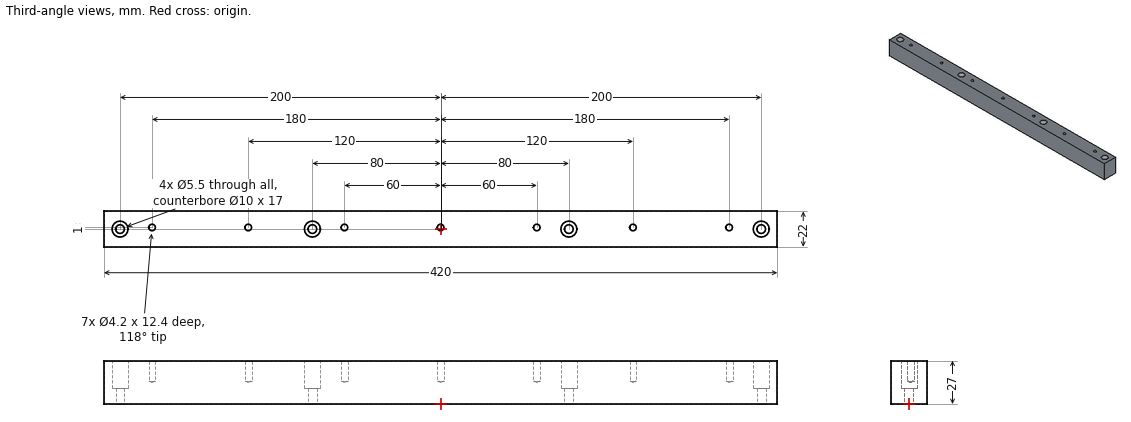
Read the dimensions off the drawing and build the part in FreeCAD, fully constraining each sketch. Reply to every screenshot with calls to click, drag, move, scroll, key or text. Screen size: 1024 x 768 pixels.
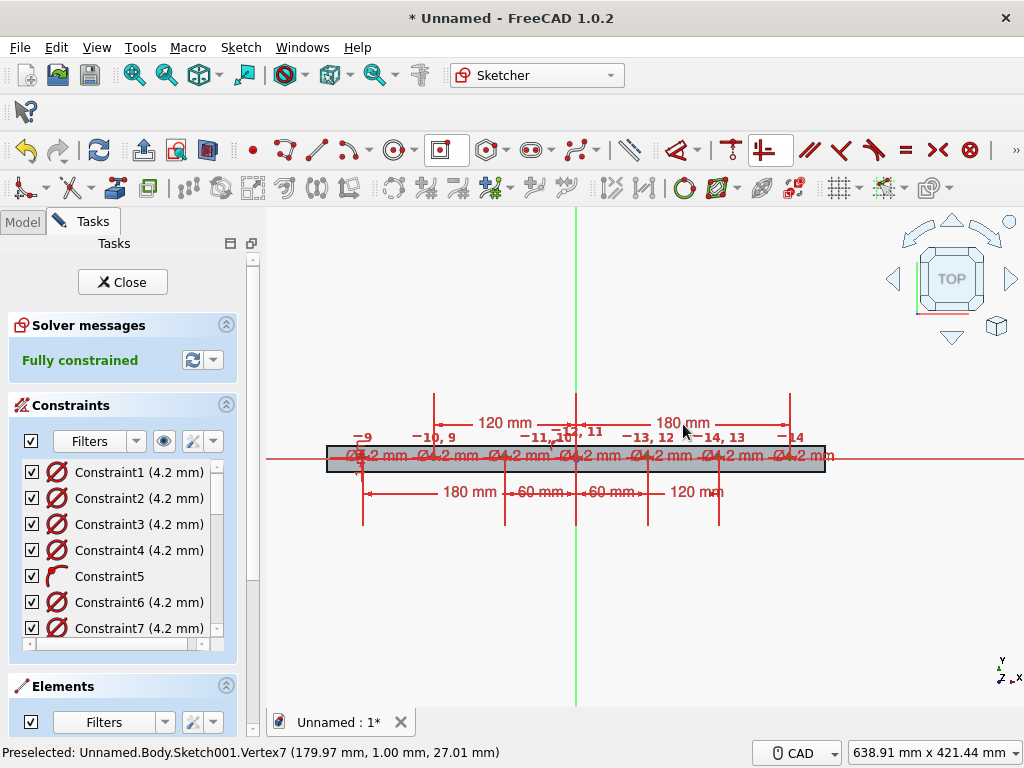
click(123, 282)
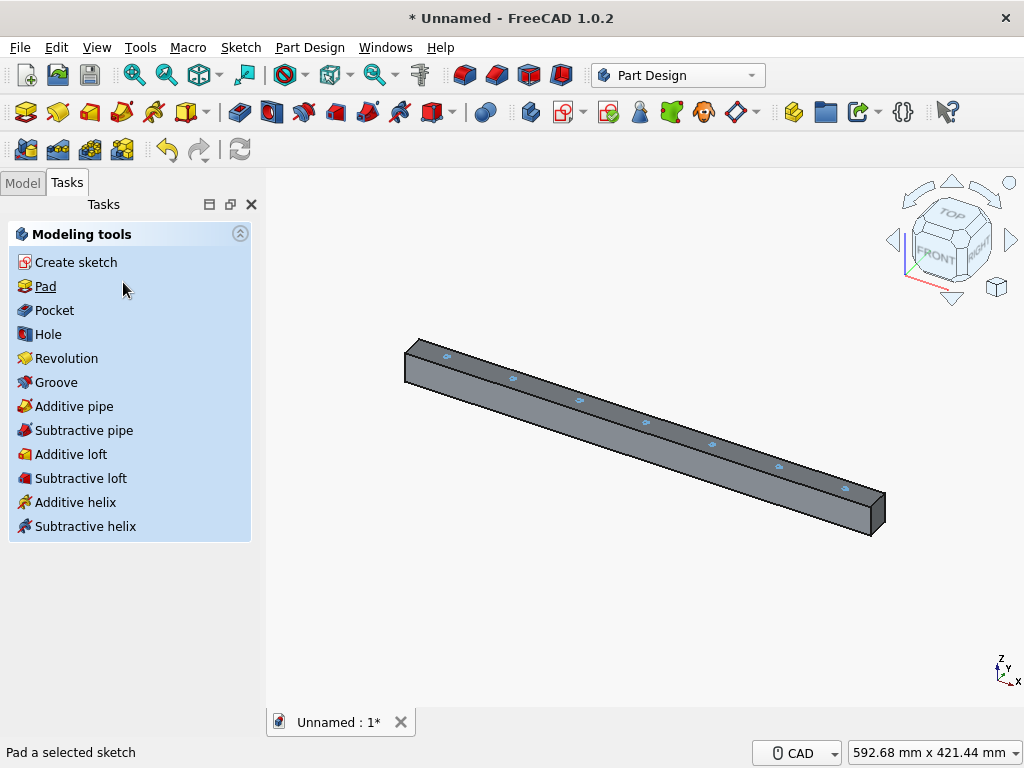
click(272, 112)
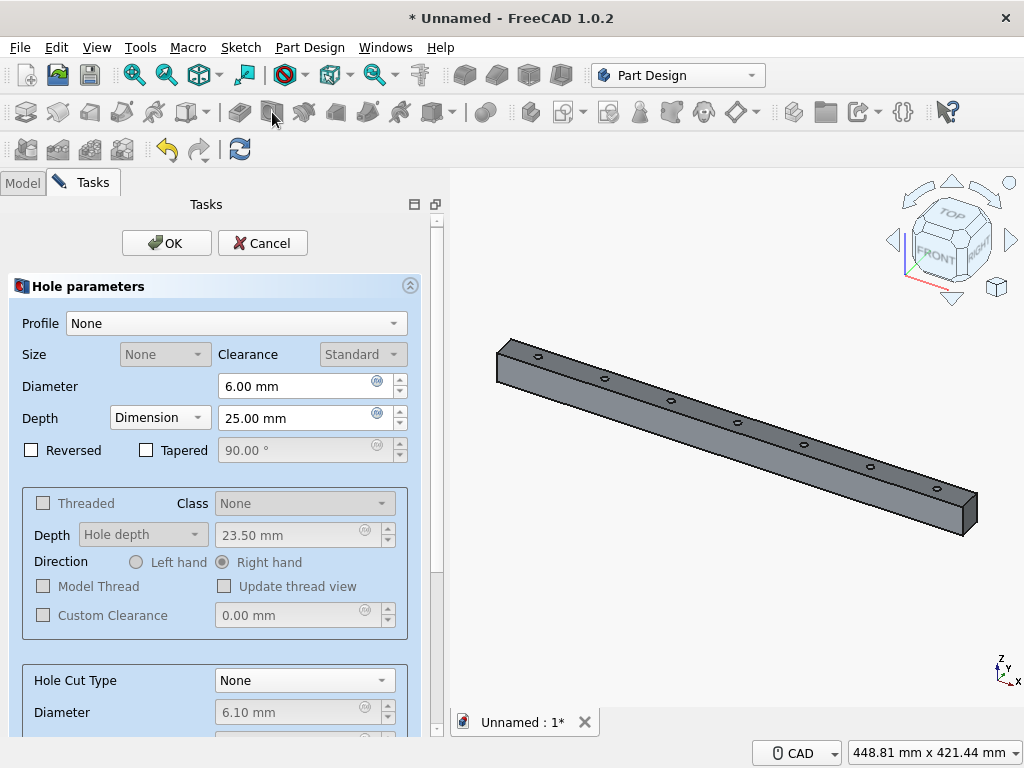
triple_click(305, 386)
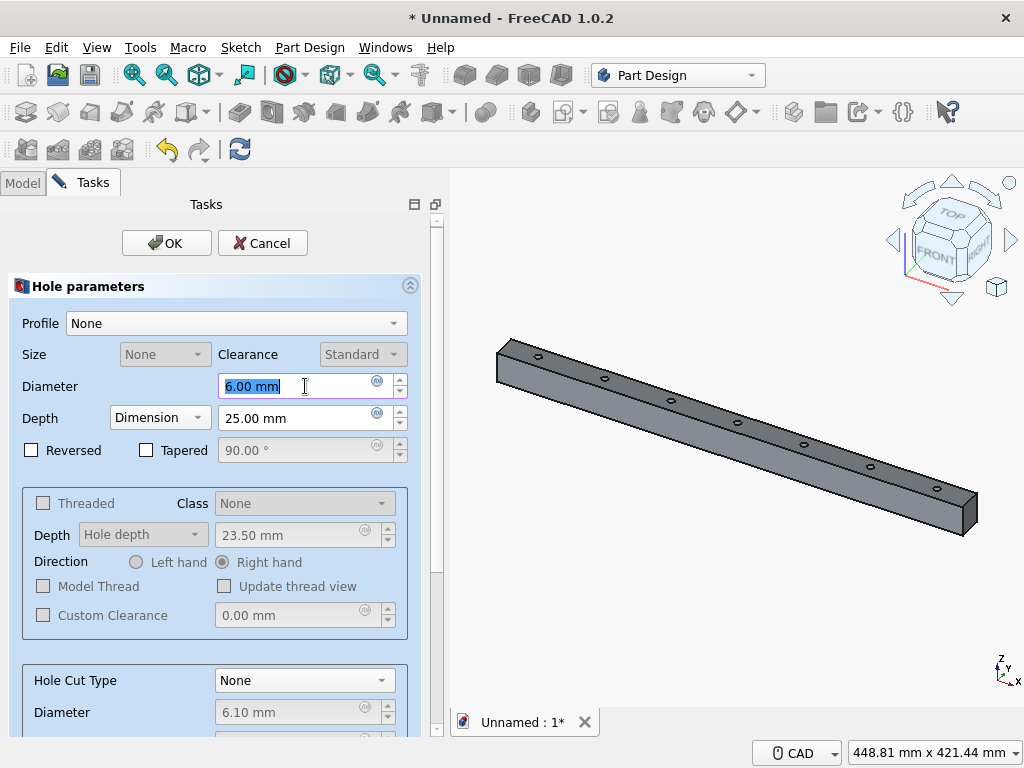
text(4.2)
key(Tab)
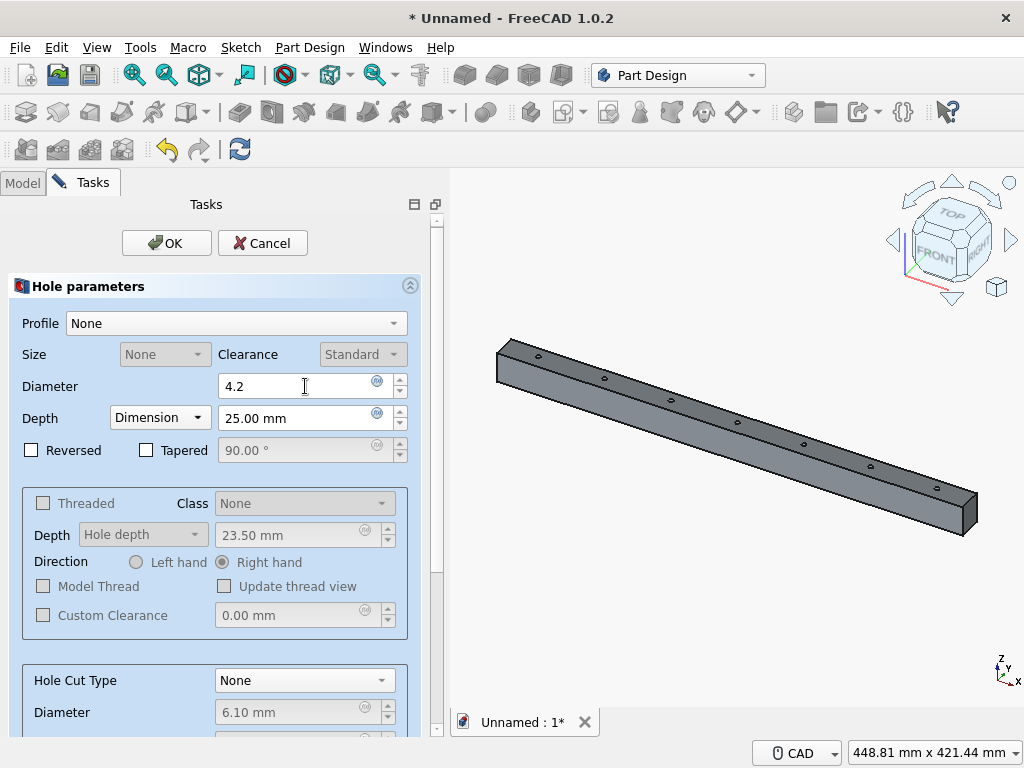
triple_click(305, 418)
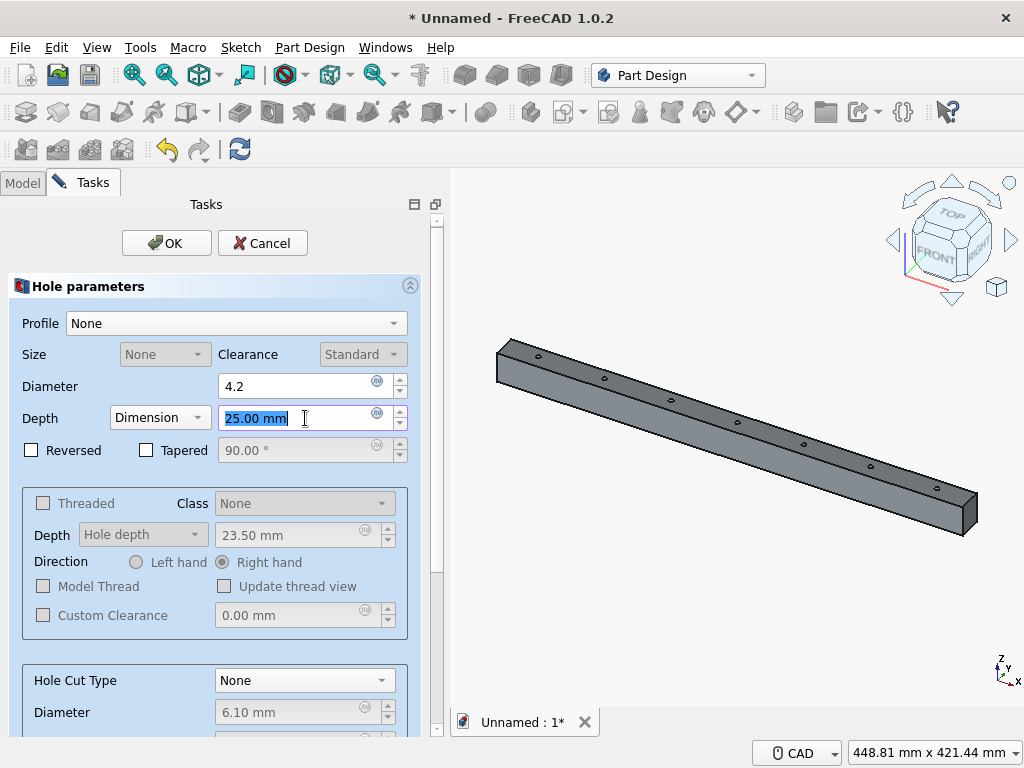
text(12.4)
key(Tab)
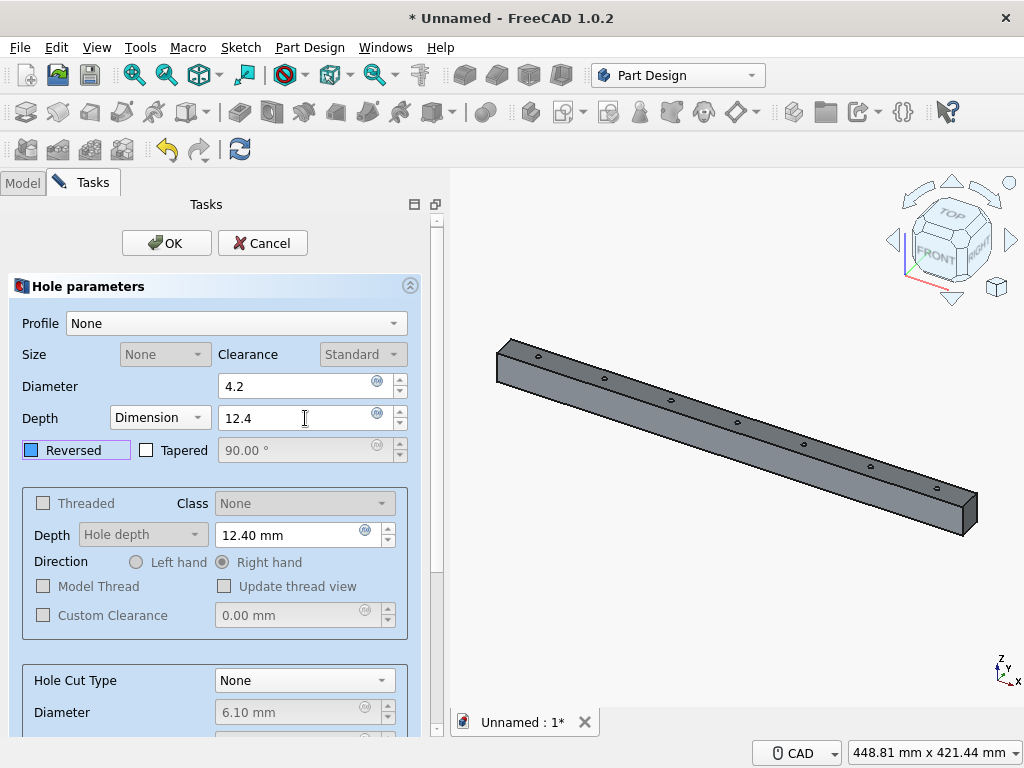
click(167, 243)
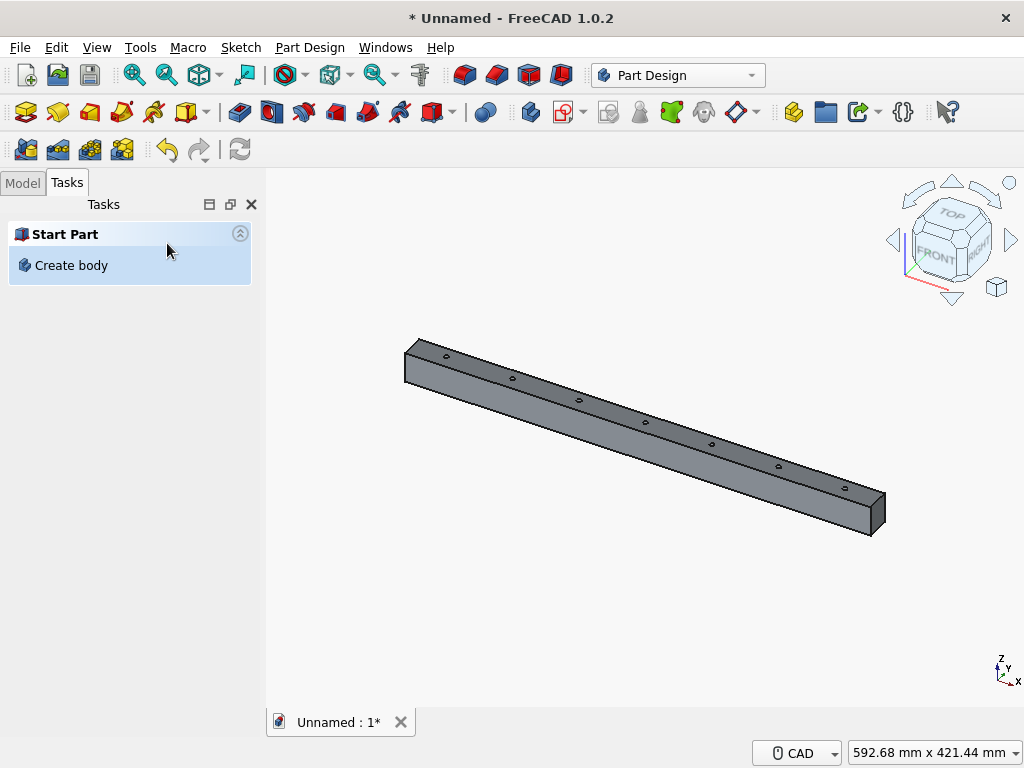
scroll(840, 492, up, 4)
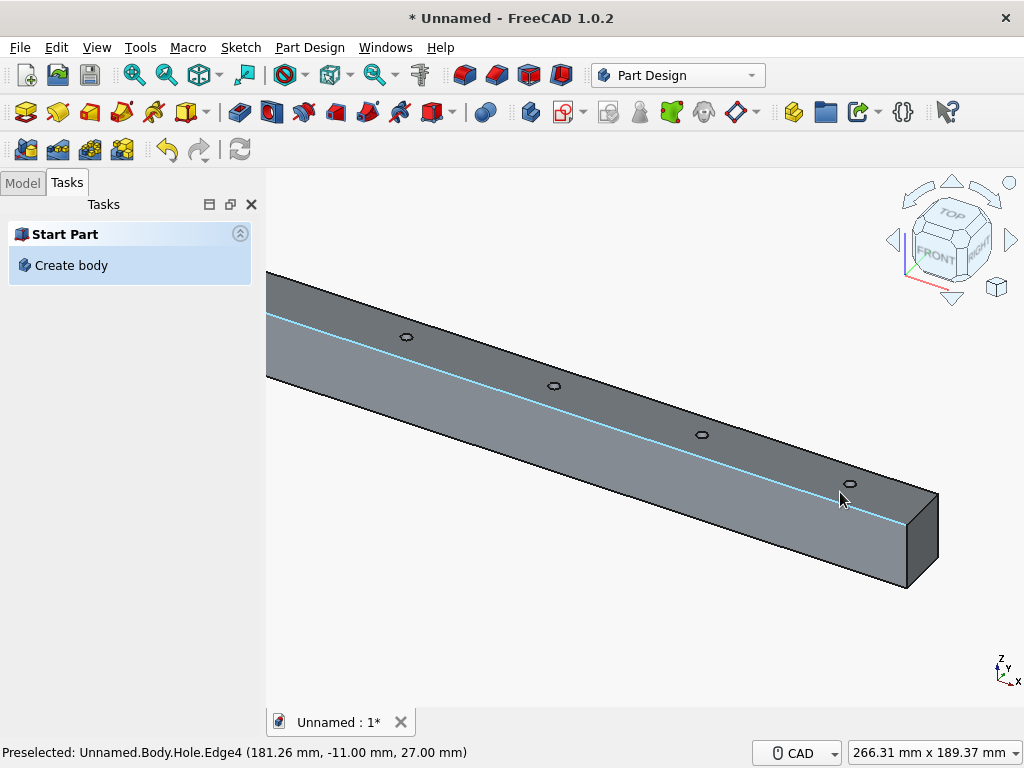
key(v)
key(f)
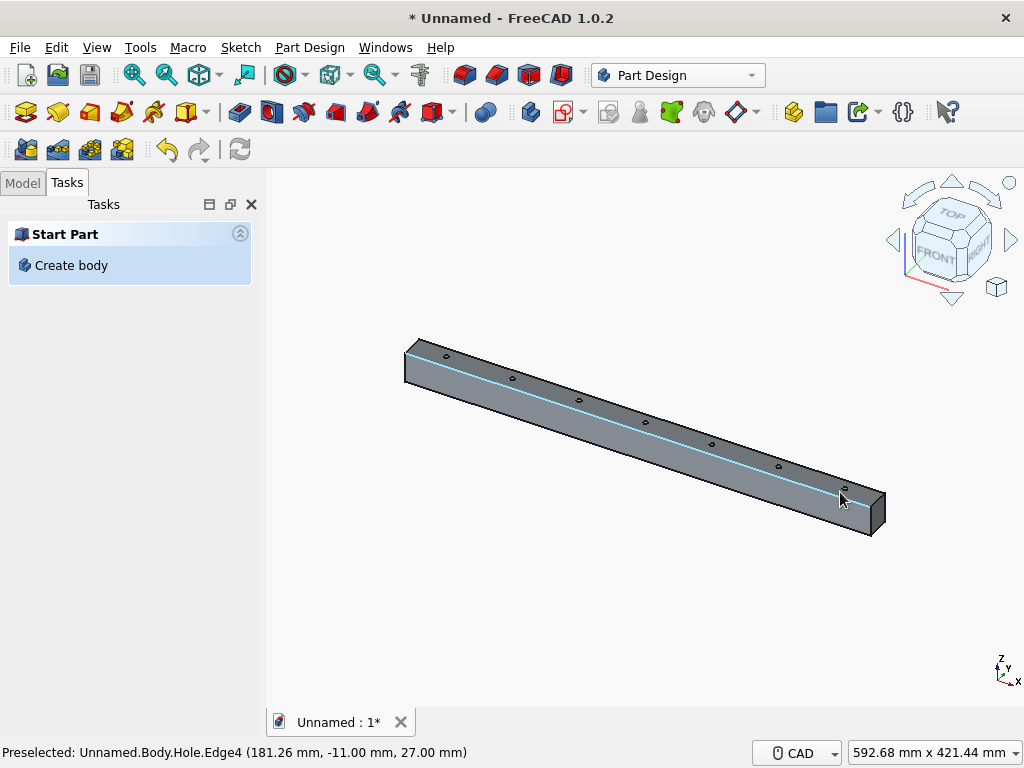
key(0)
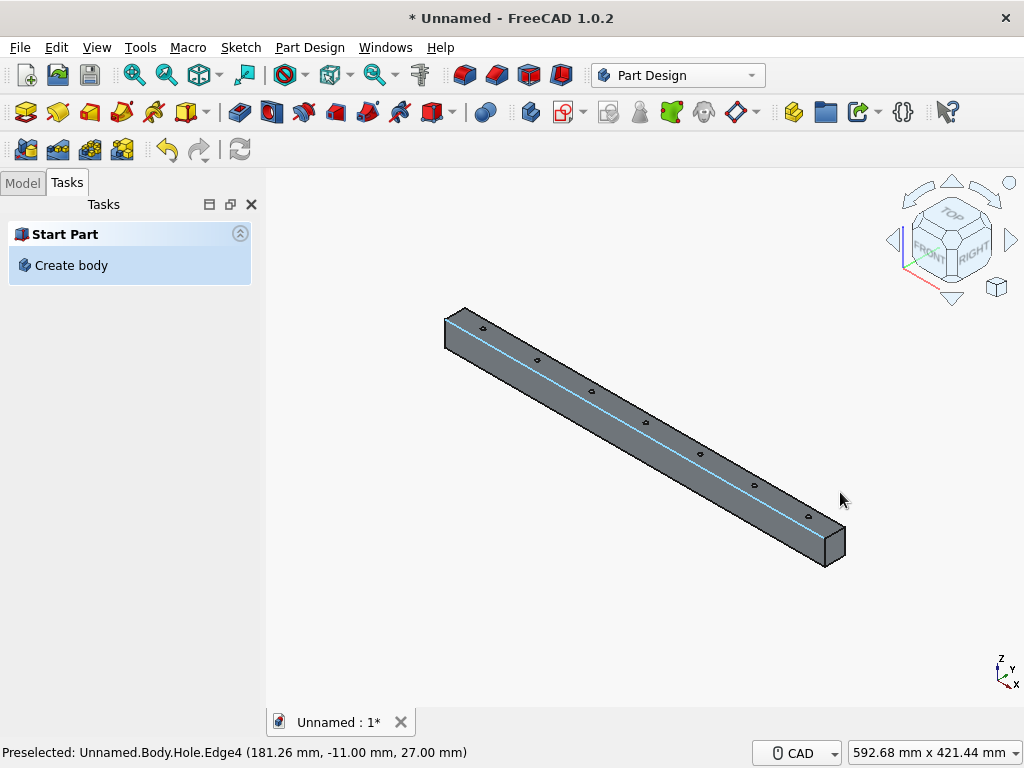
scroll(802, 520, up, 4)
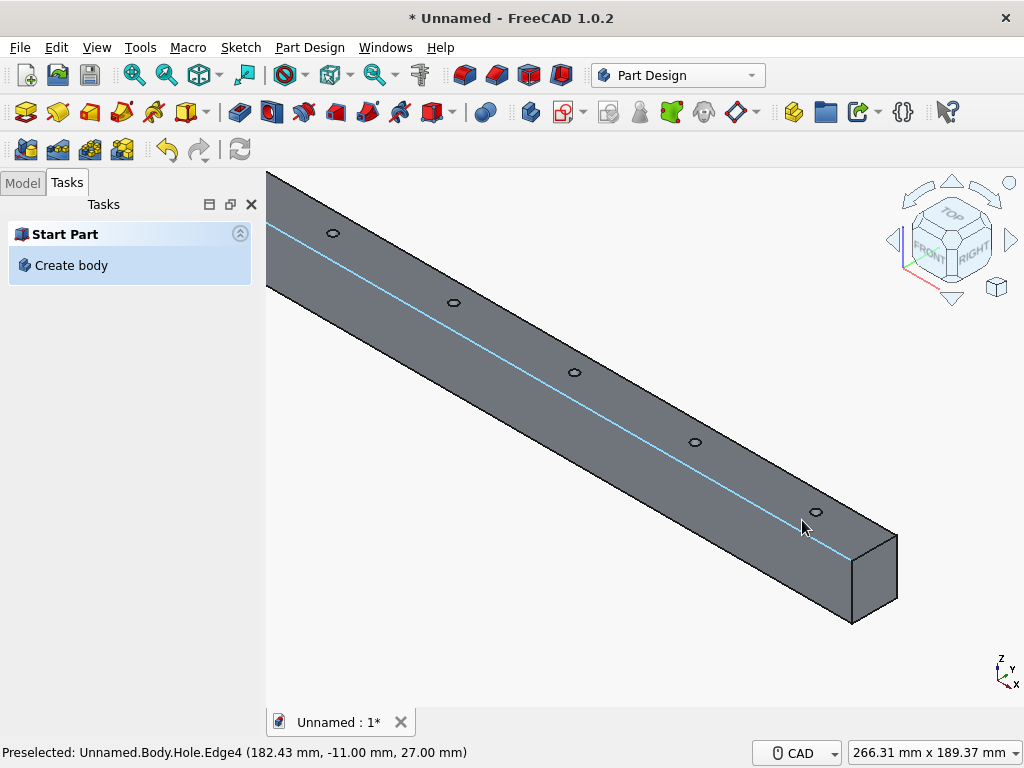
click(681, 450)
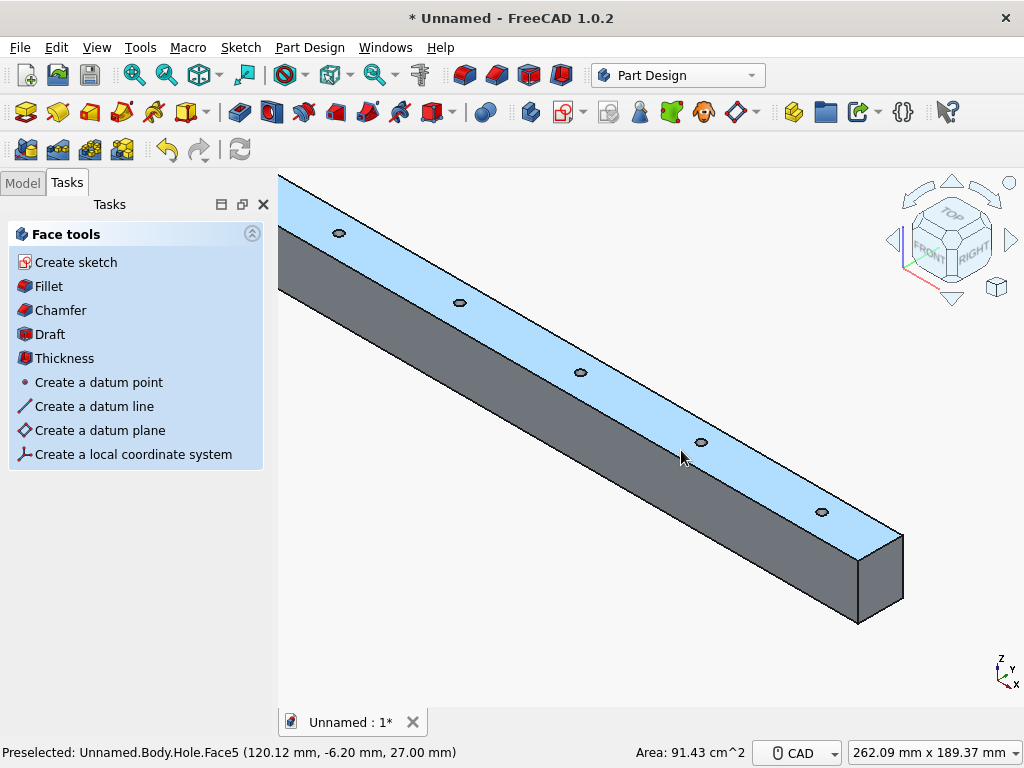
click(564, 112)